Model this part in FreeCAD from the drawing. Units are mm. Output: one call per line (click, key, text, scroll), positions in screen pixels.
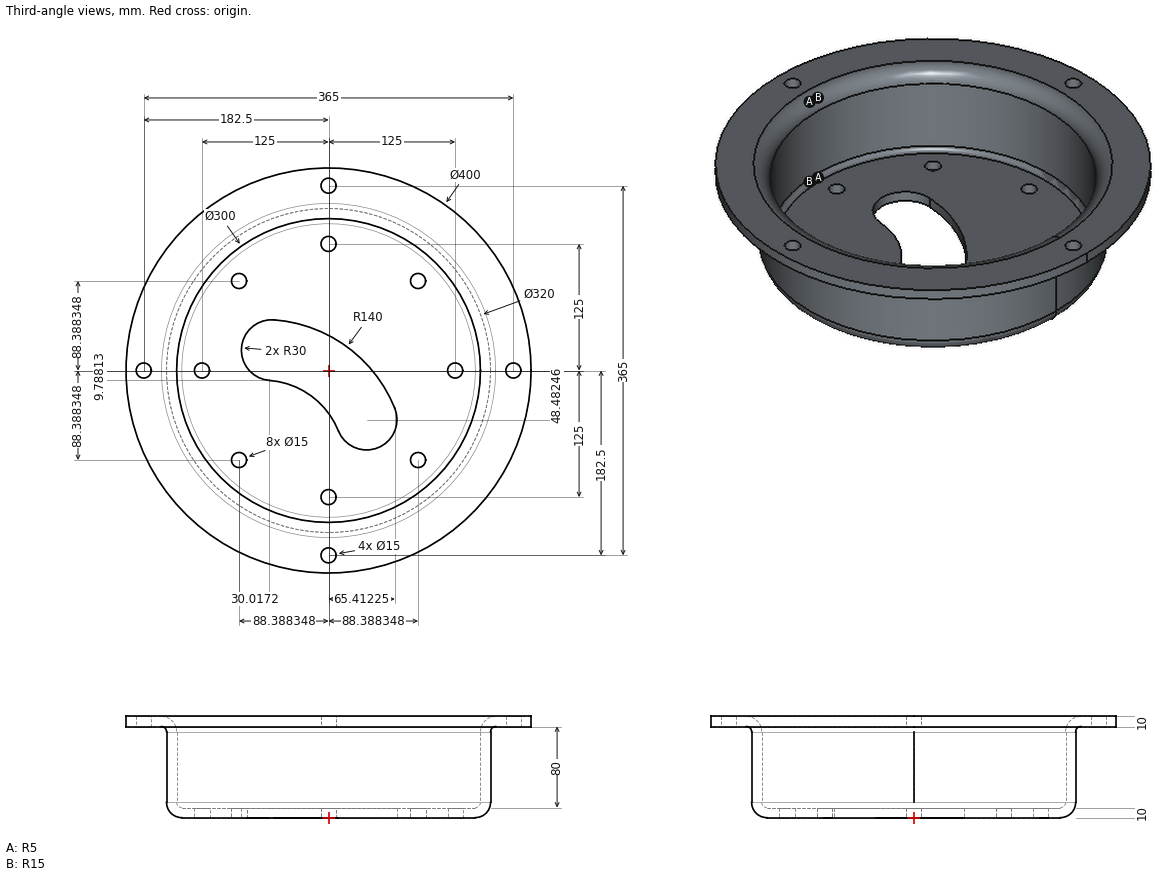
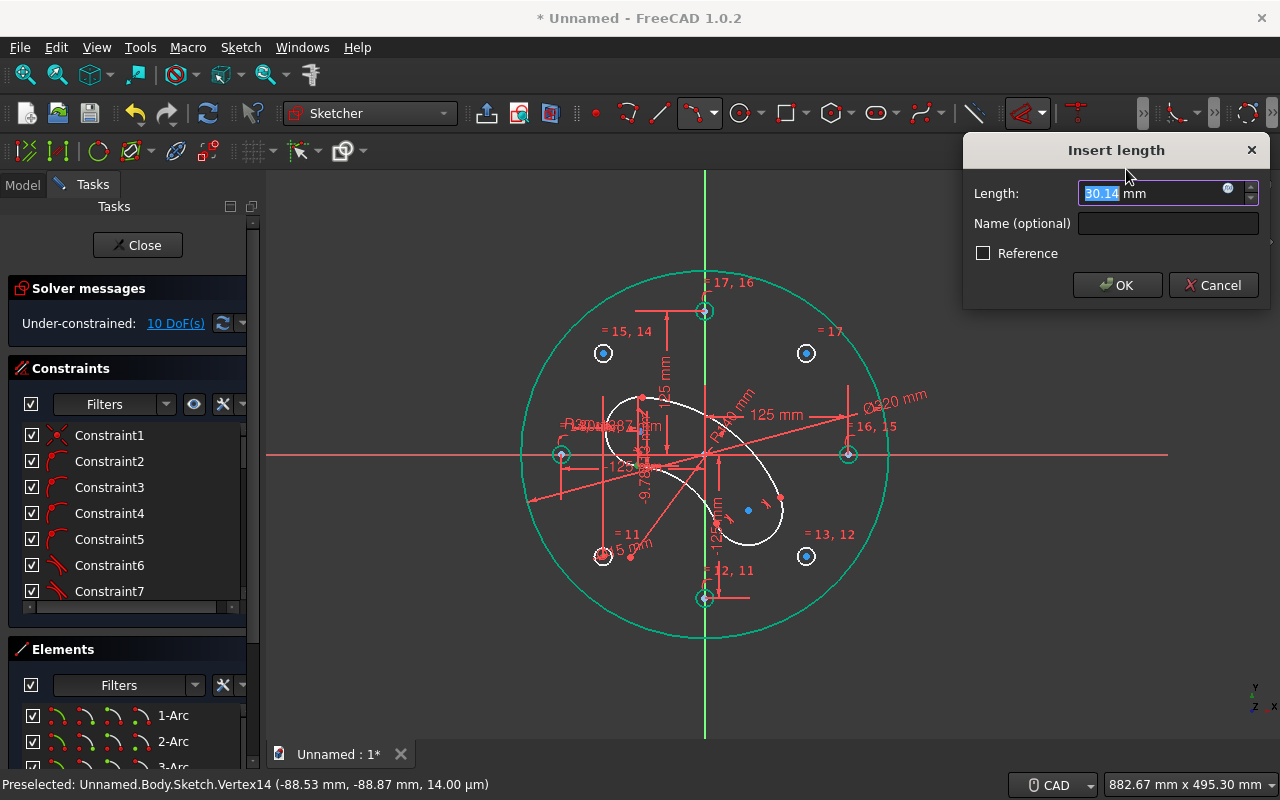
text(30.0172)
key(Return)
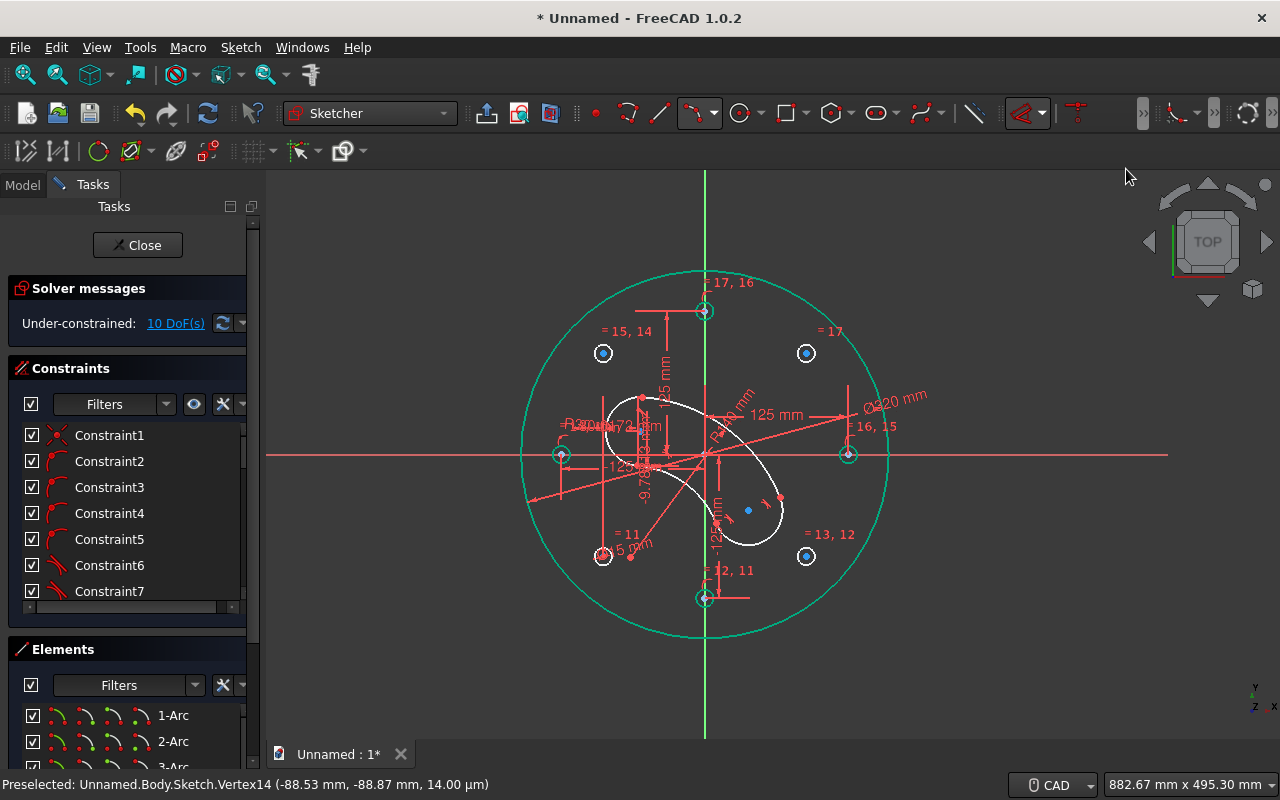
click(638, 466)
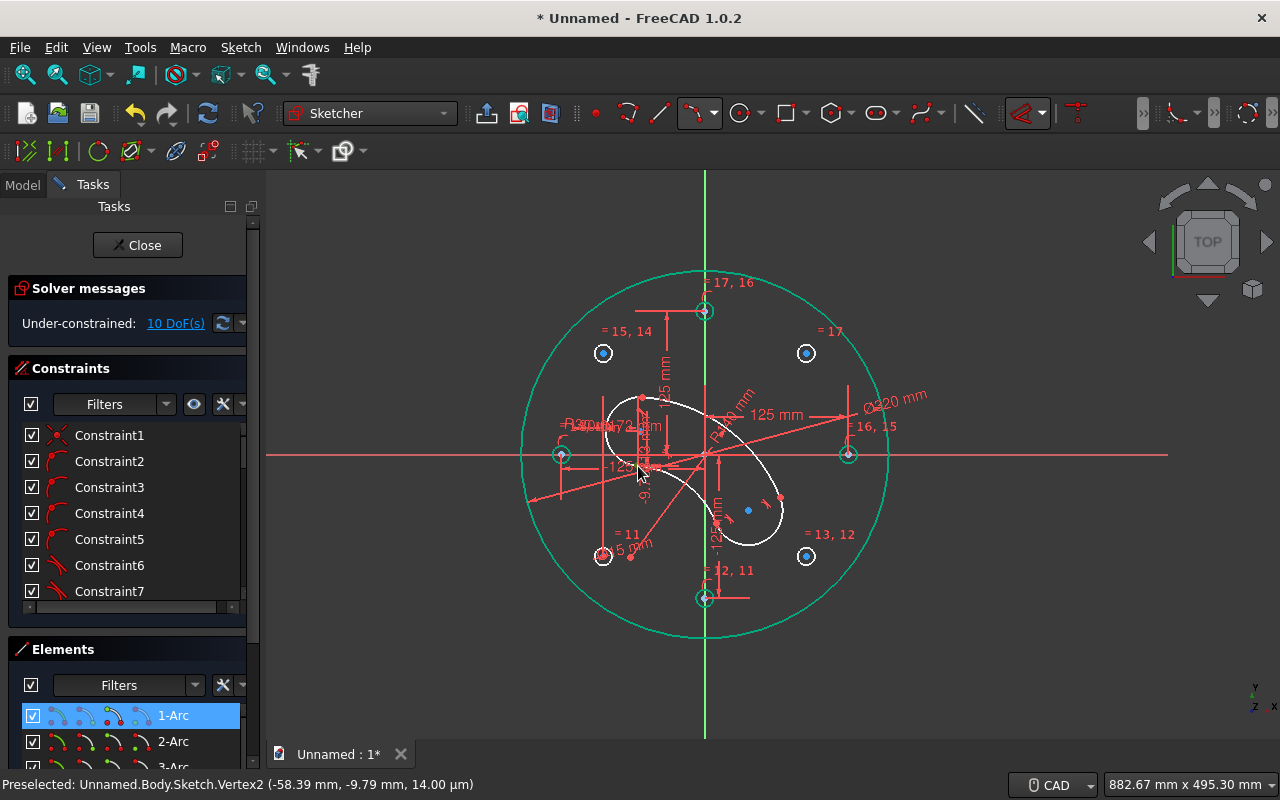
click(603, 353)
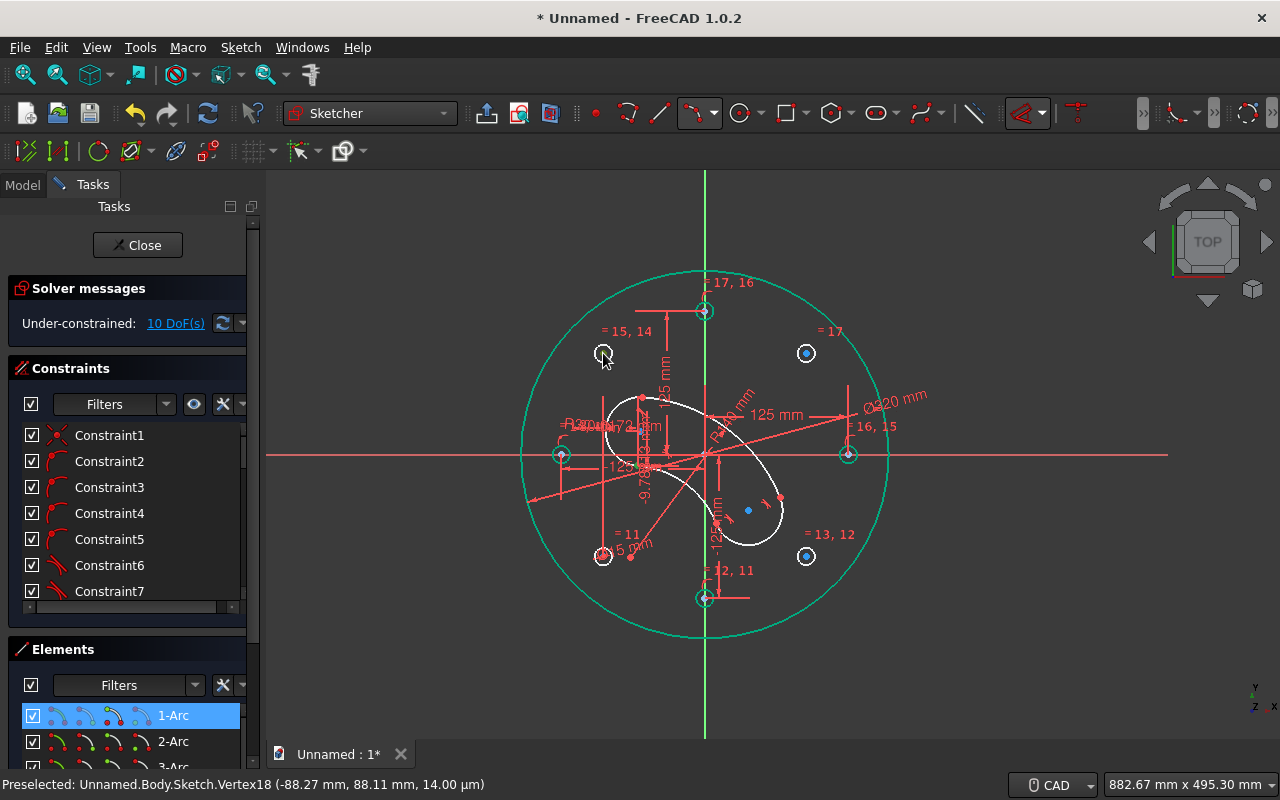
key(l)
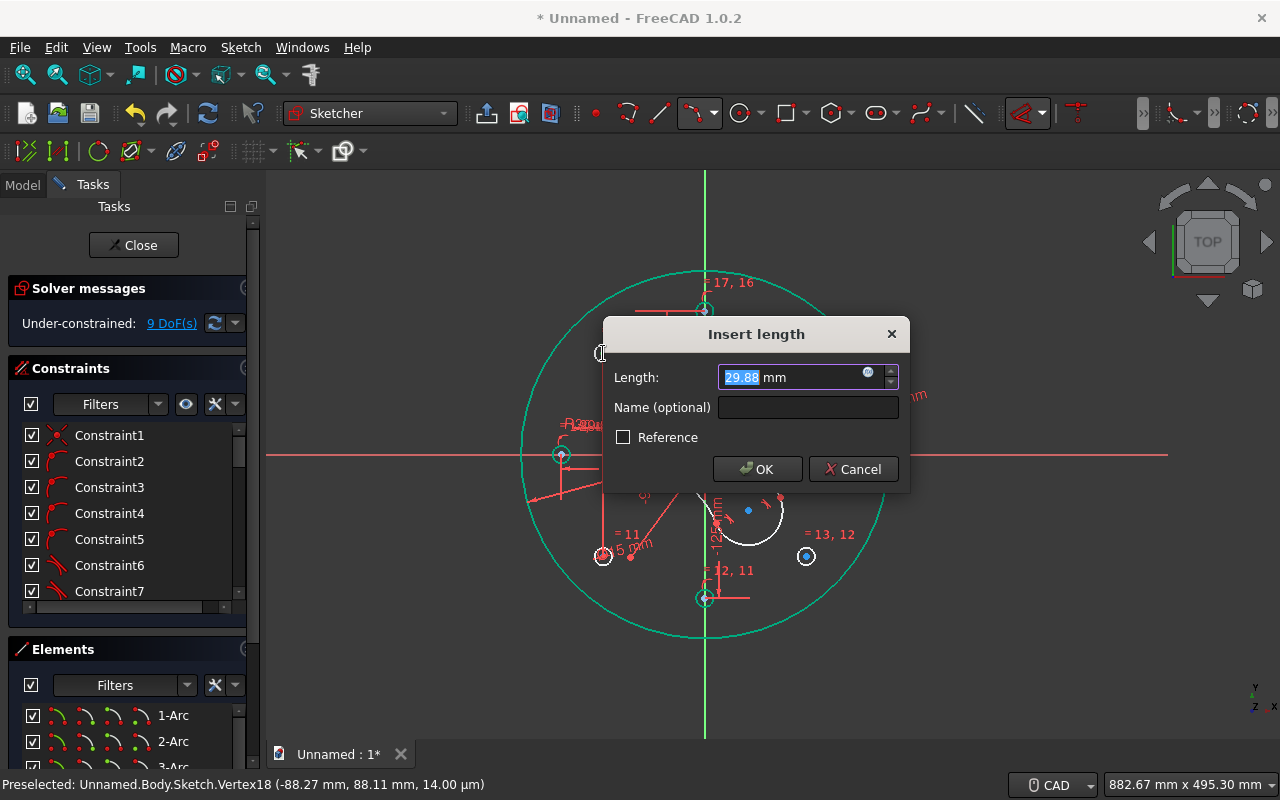
text(30.0172)
key(Return)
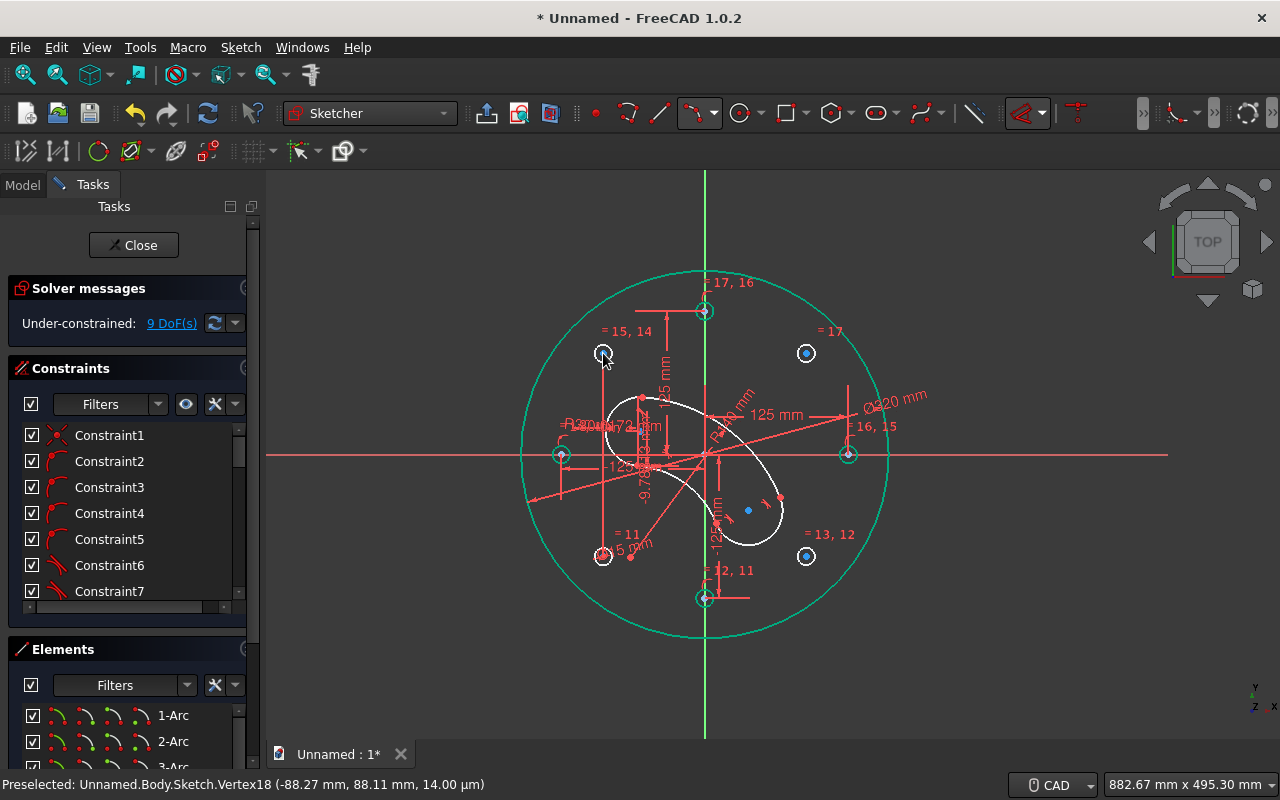
click(780, 498)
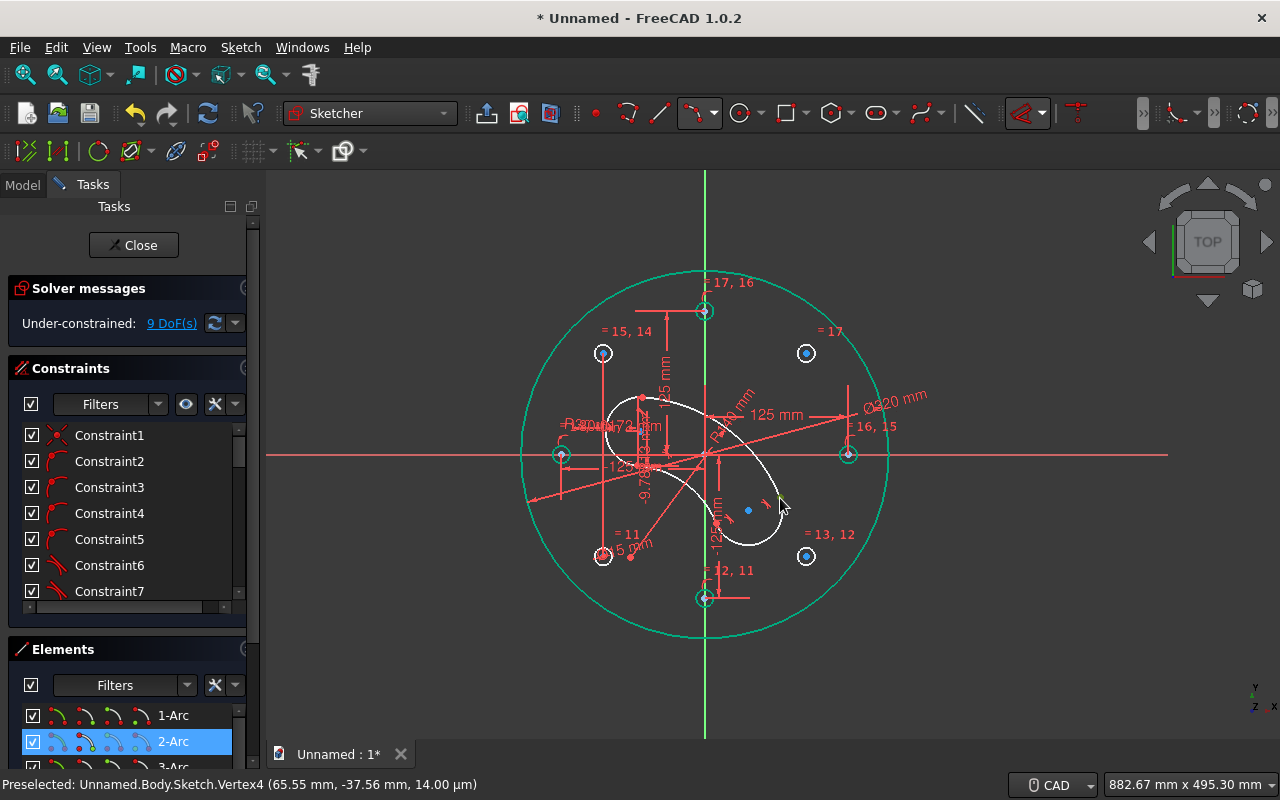
key(l)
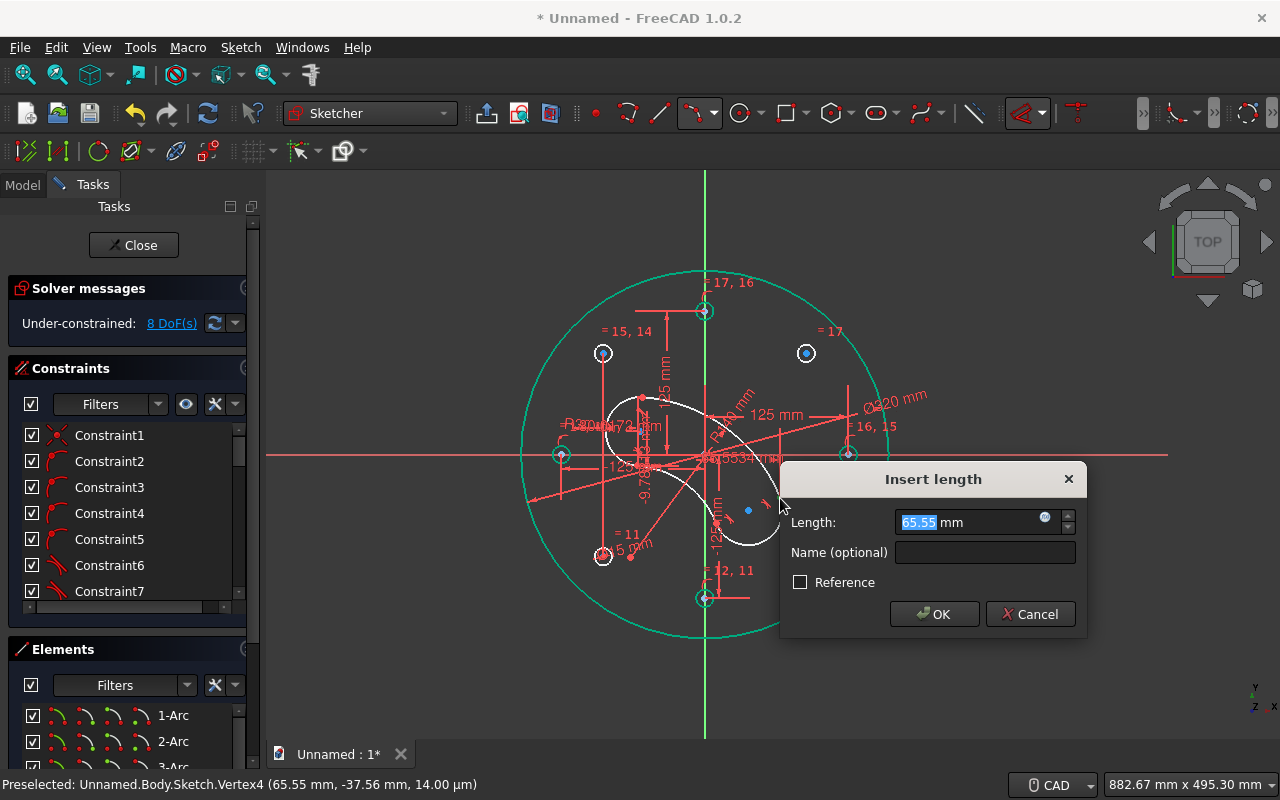
text(65.41225)
key(Return)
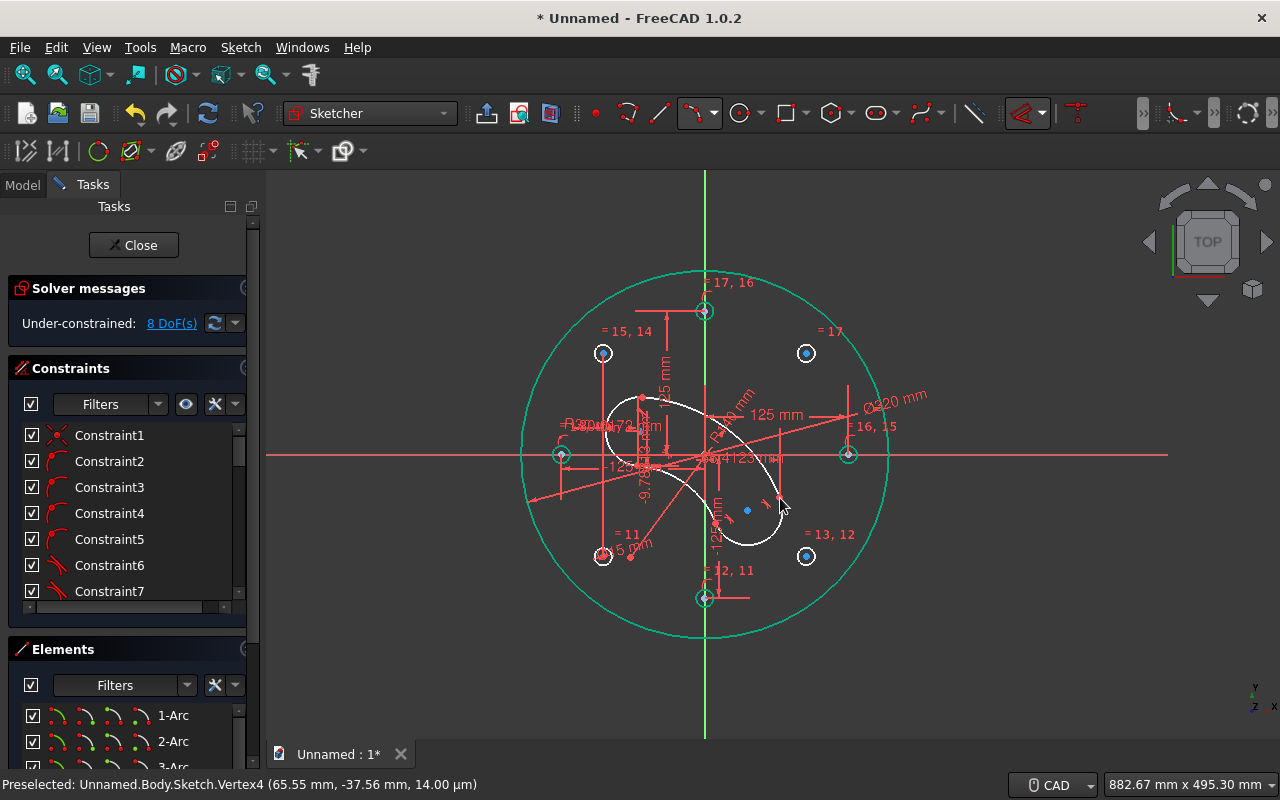
click(748, 511)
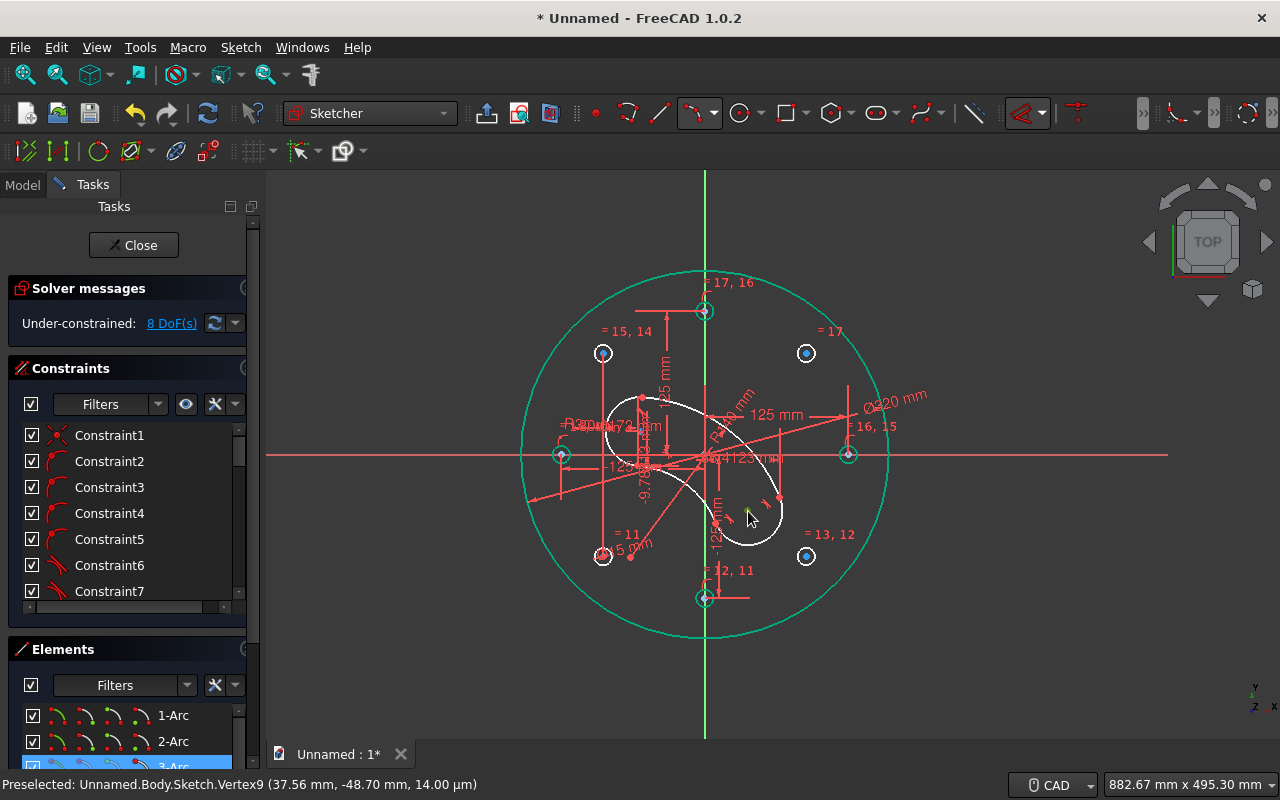
click(1044, 114)